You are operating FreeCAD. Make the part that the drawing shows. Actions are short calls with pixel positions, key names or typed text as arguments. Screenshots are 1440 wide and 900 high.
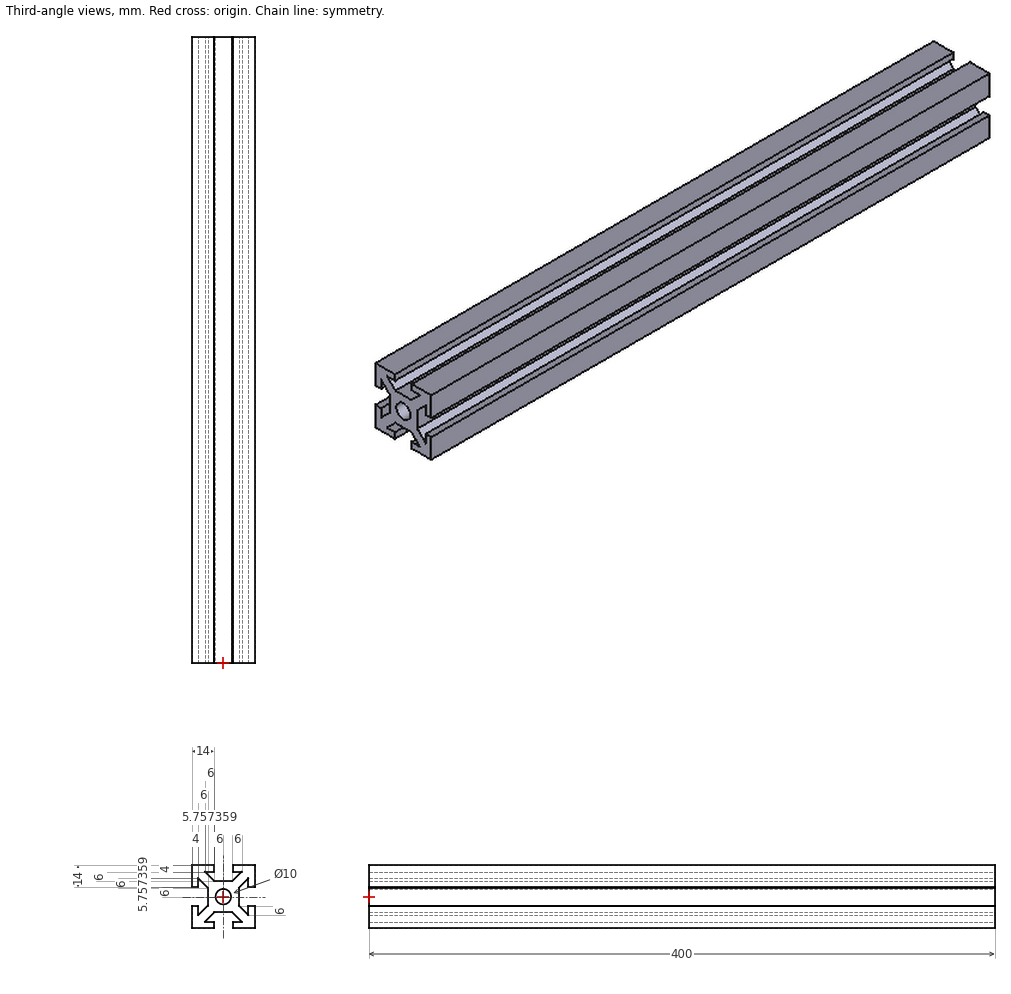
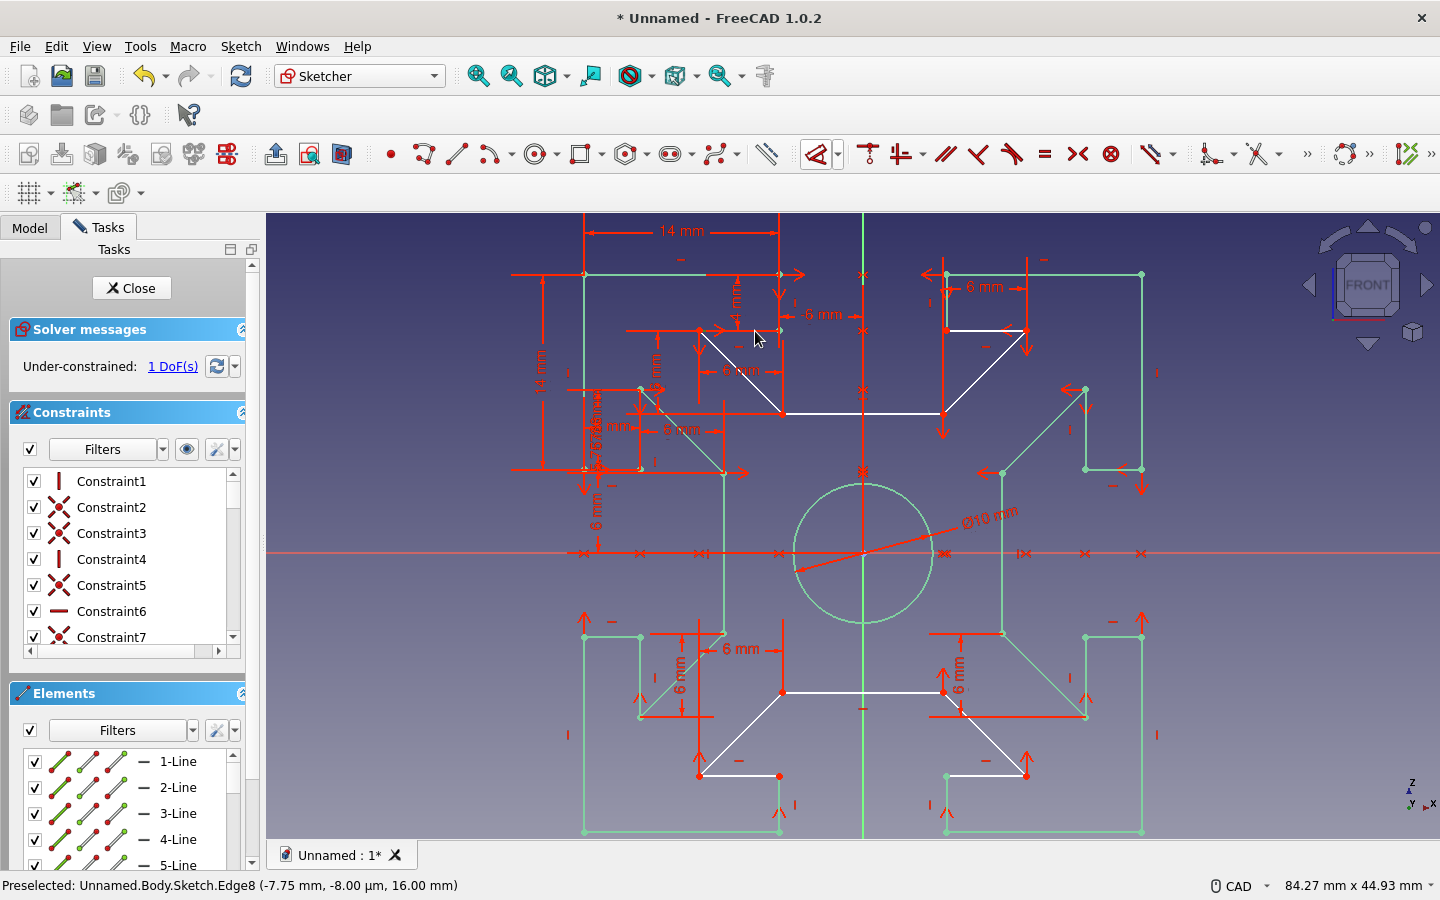
key(l)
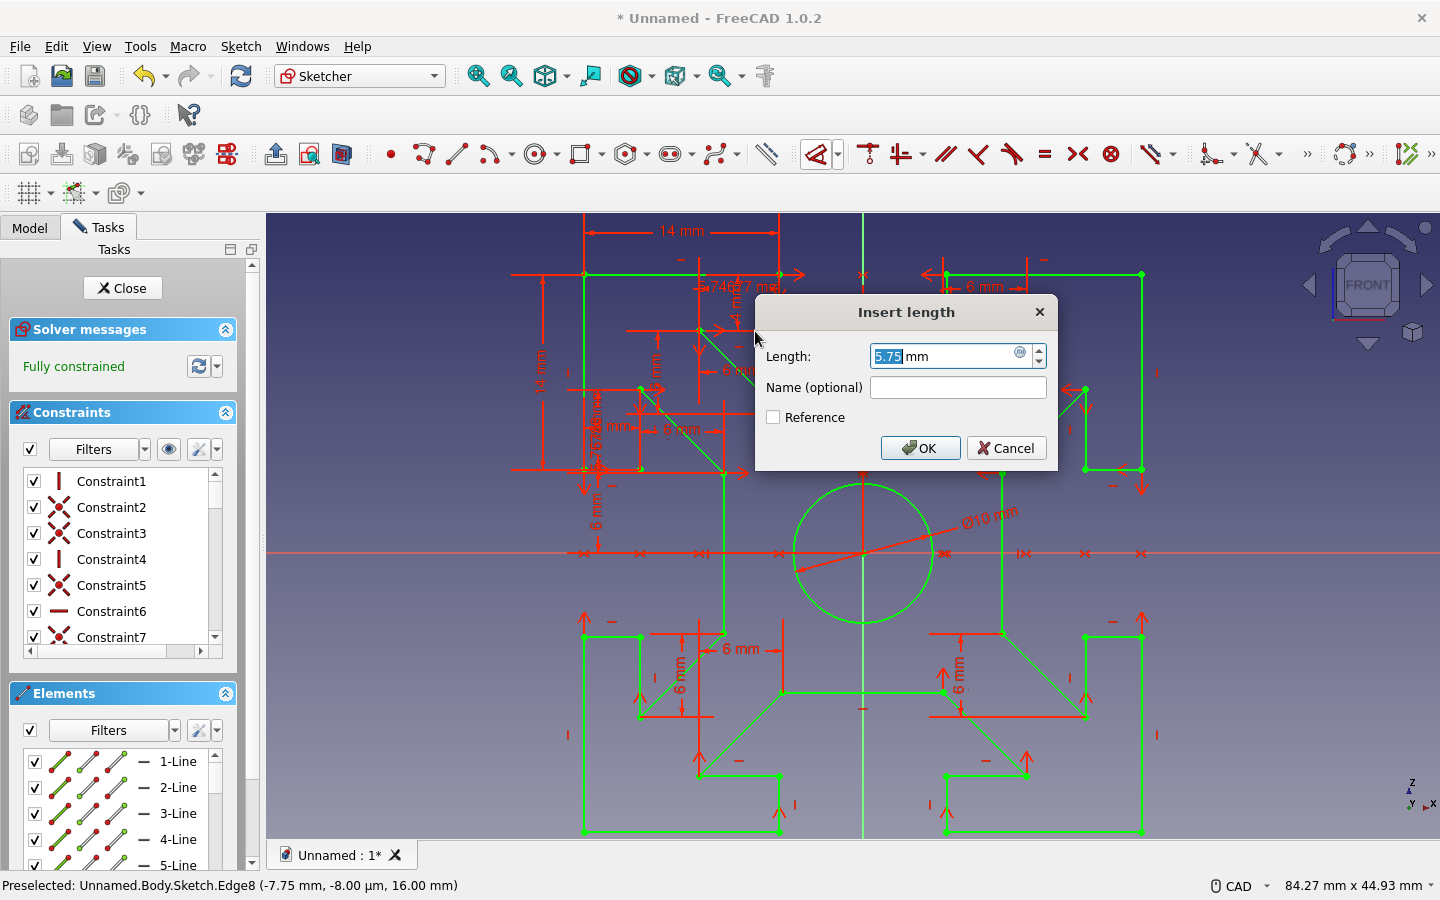
text(5.757359)
key(Return)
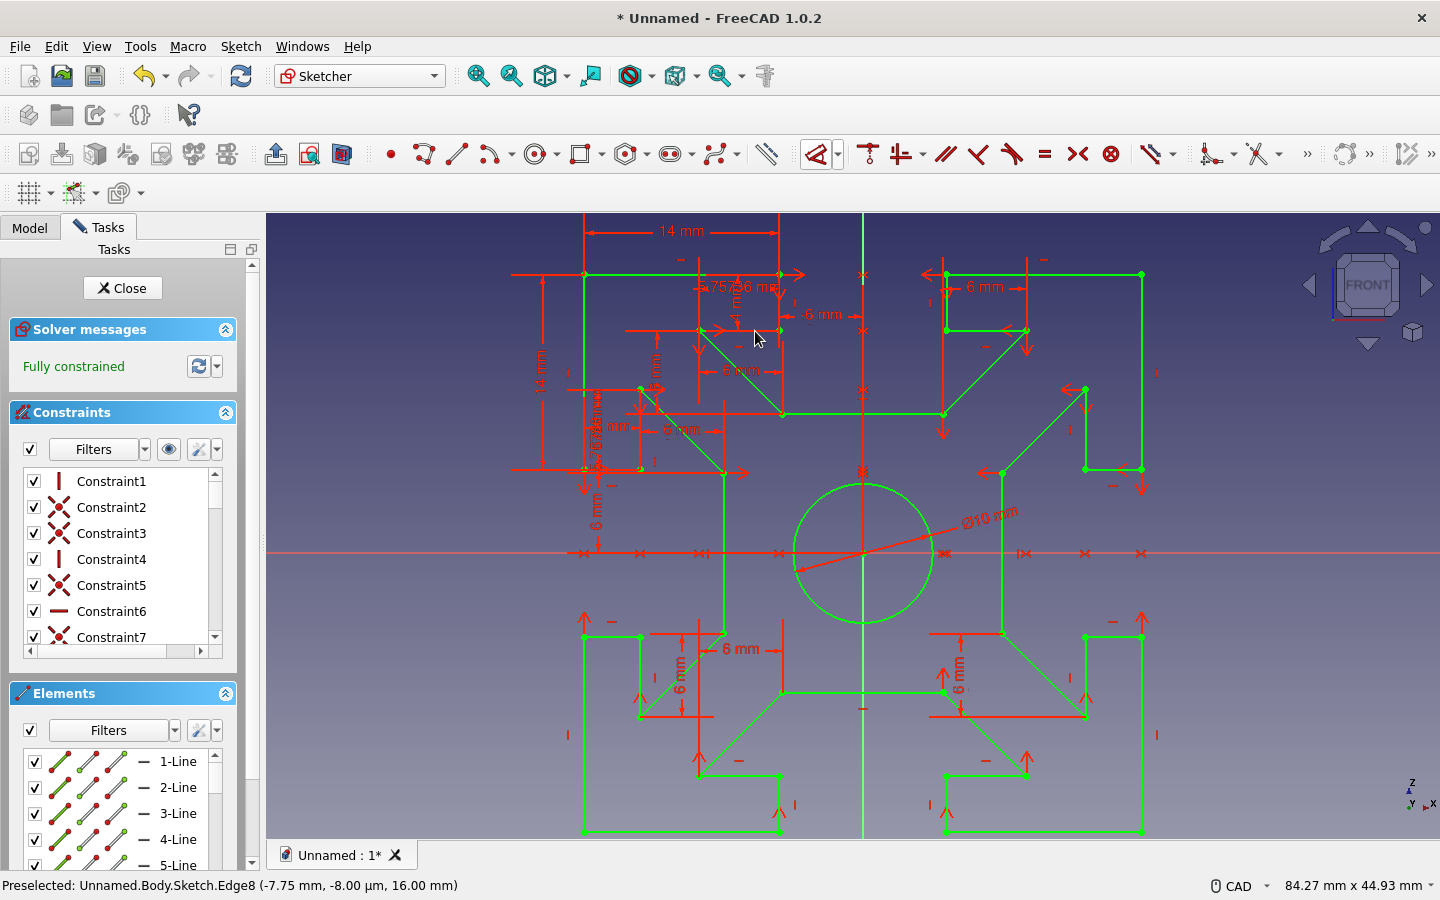
click(123, 288)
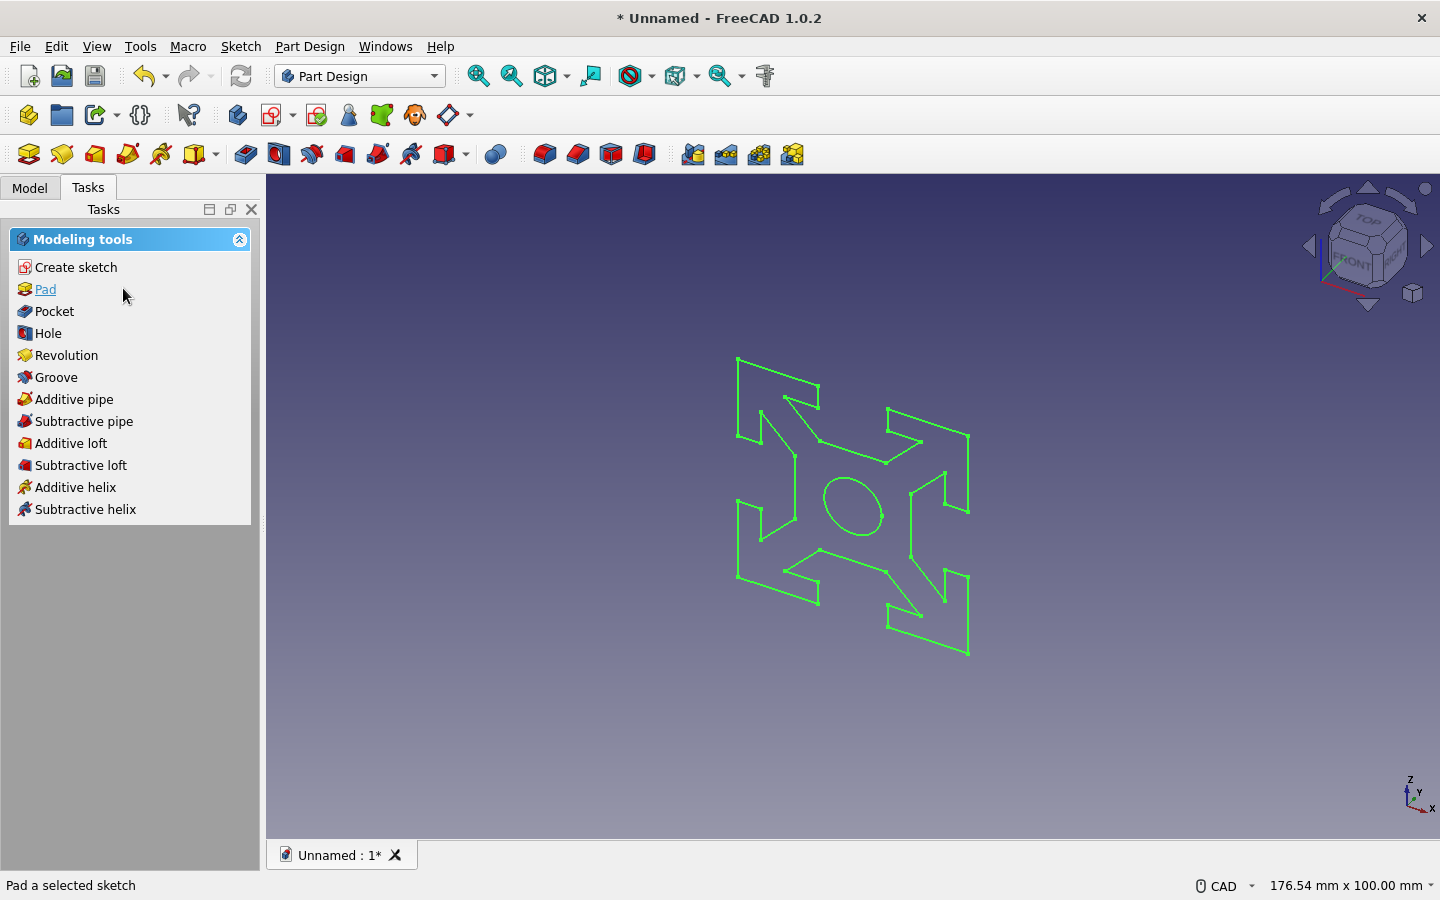
click(29, 154)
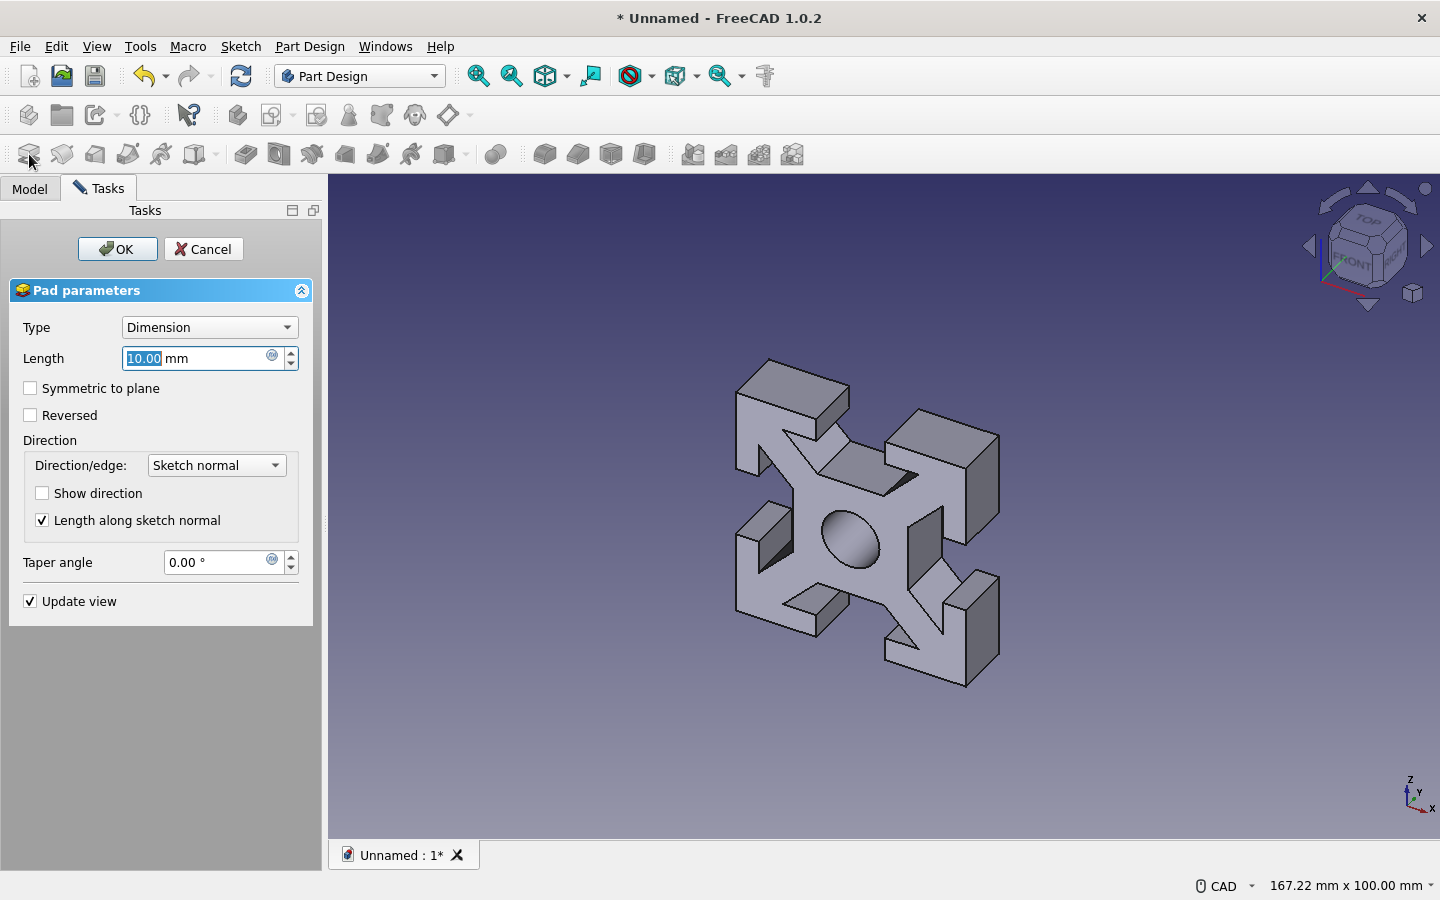
text(400)
key(Tab)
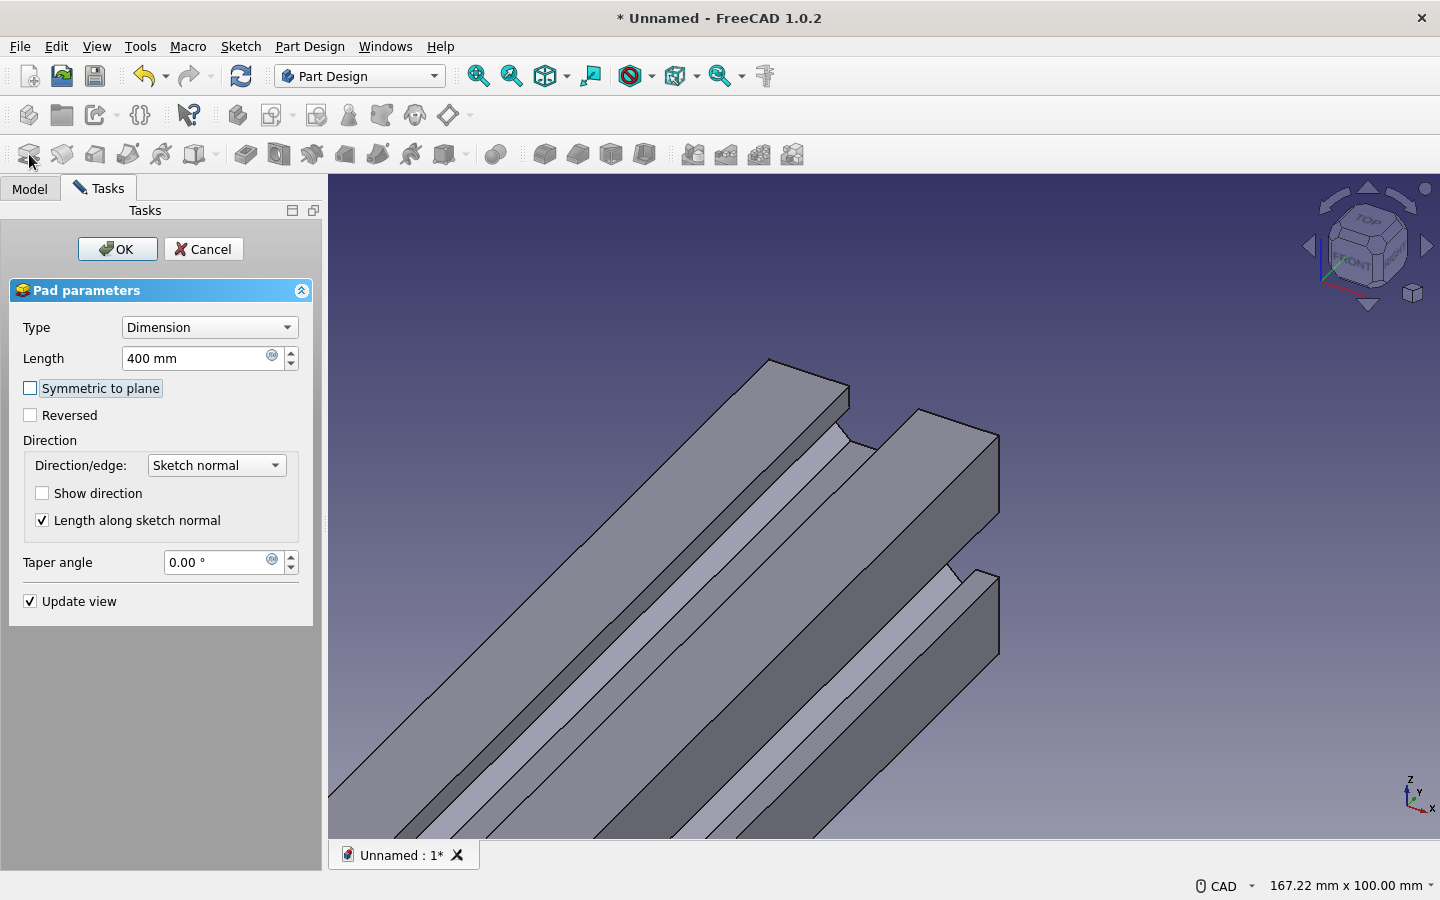
click(31, 415)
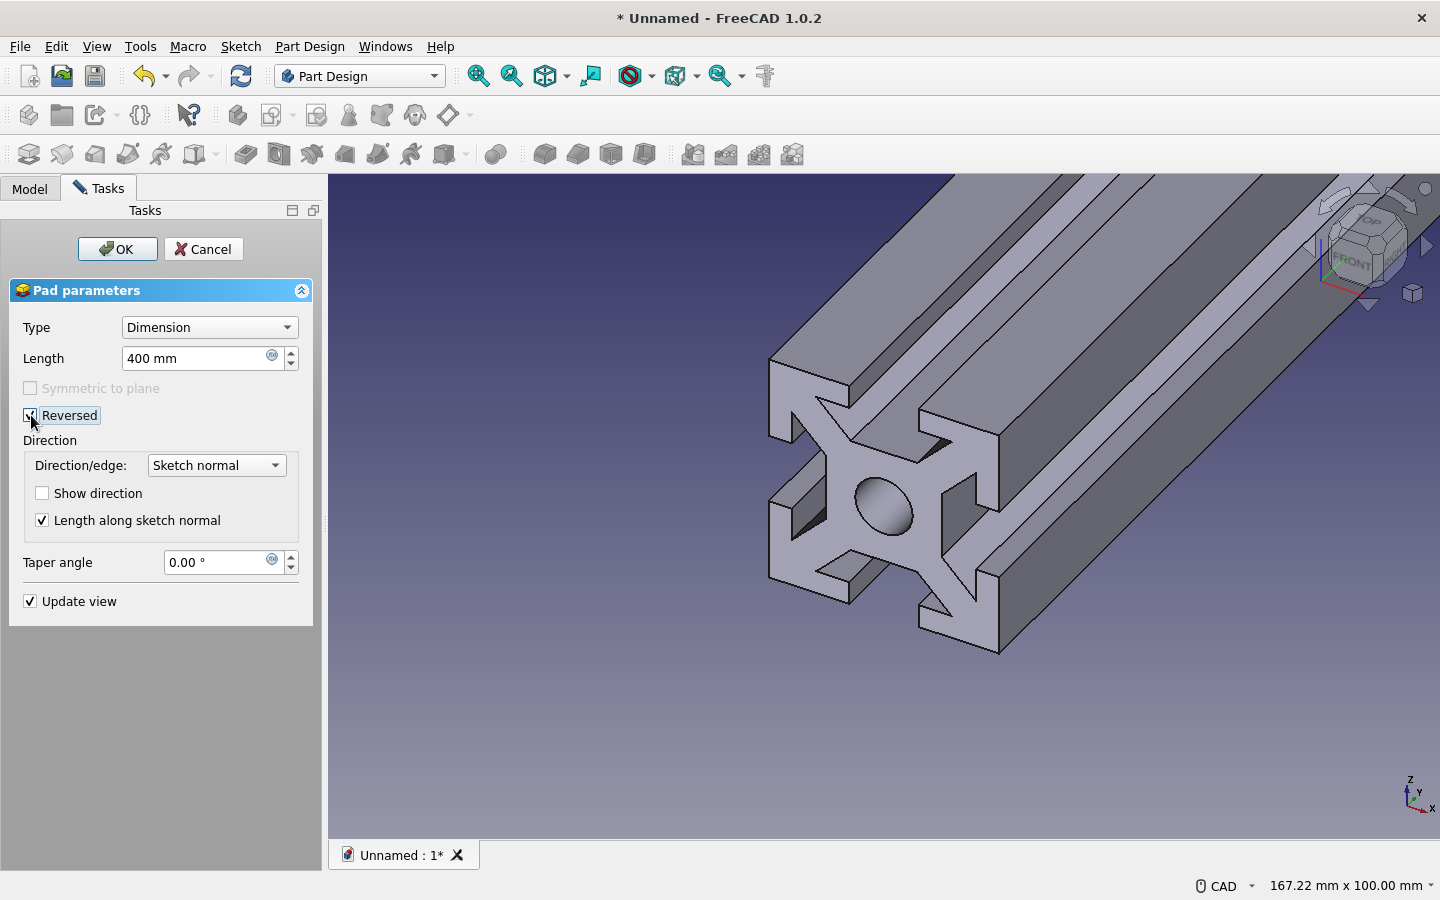
click(118, 249)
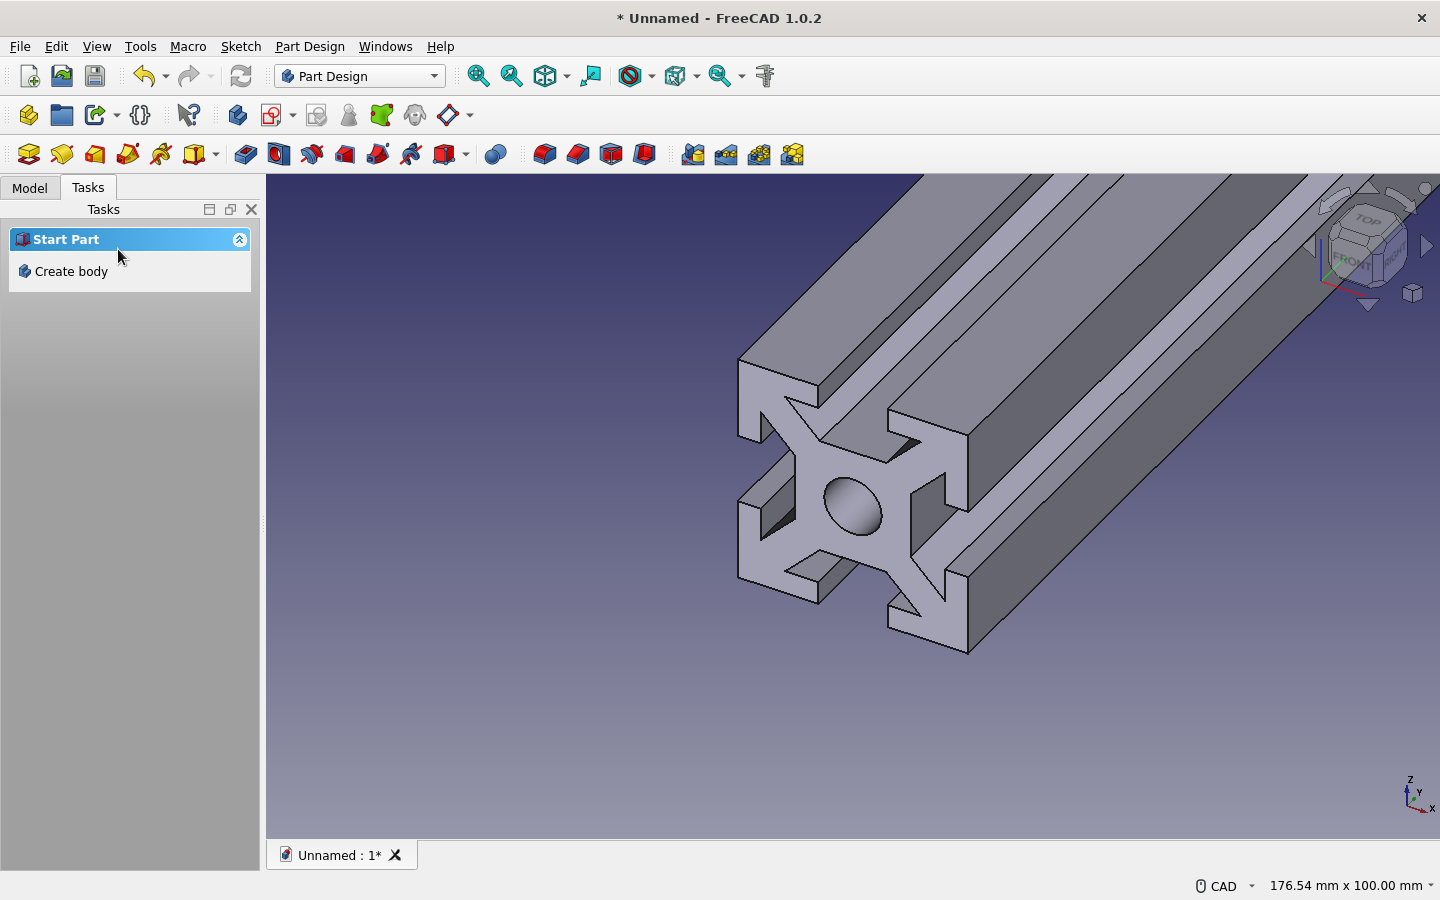
key(0)